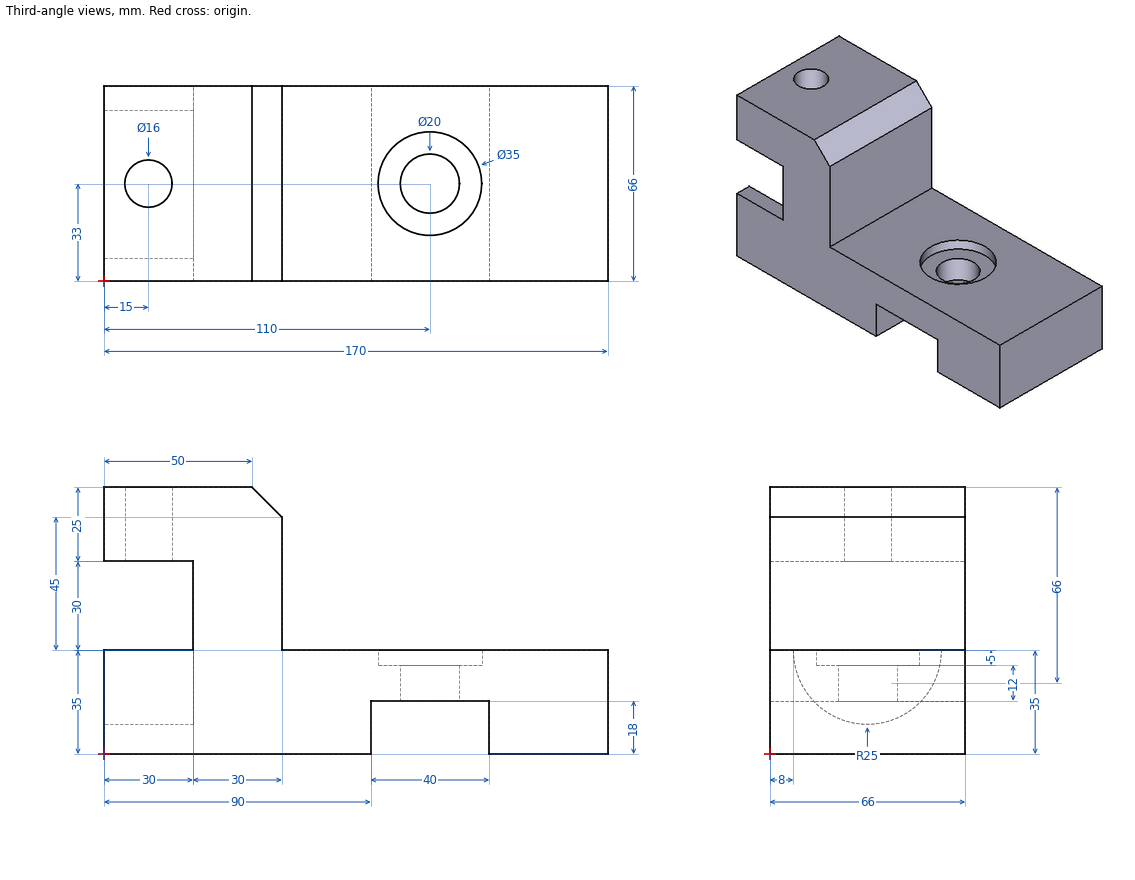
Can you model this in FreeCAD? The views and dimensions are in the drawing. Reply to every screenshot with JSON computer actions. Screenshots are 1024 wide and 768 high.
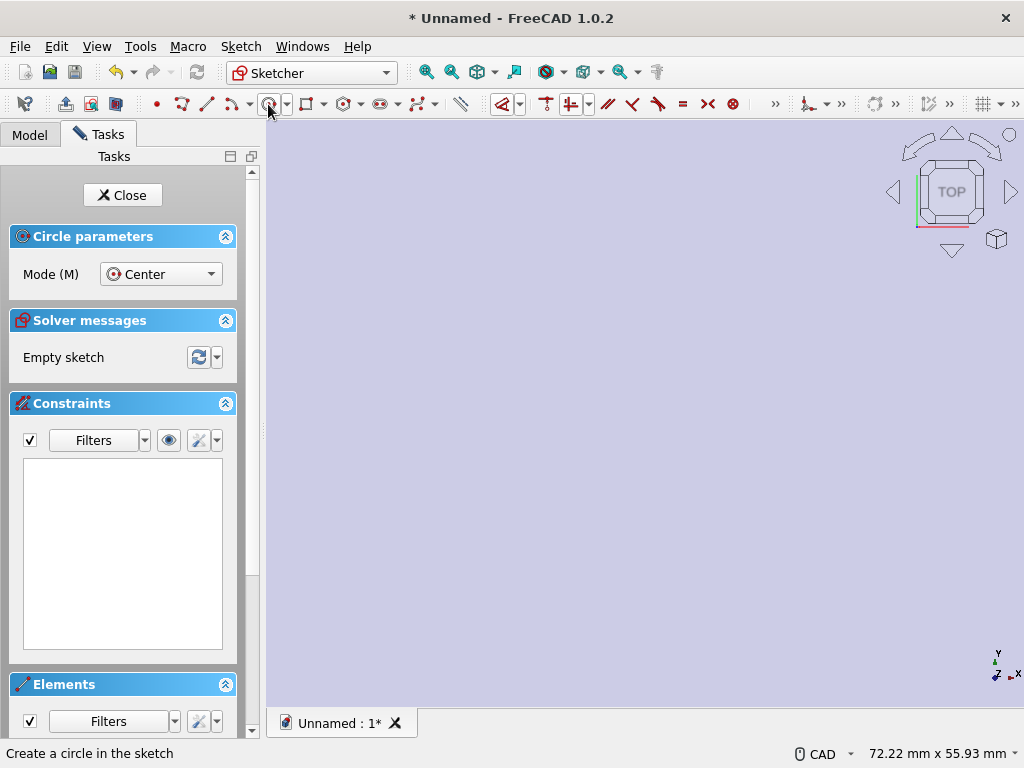
{"action": "left_click", "coordinate": [574, 411]}
{"action": "mouse_move", "coordinate": [704, 281]}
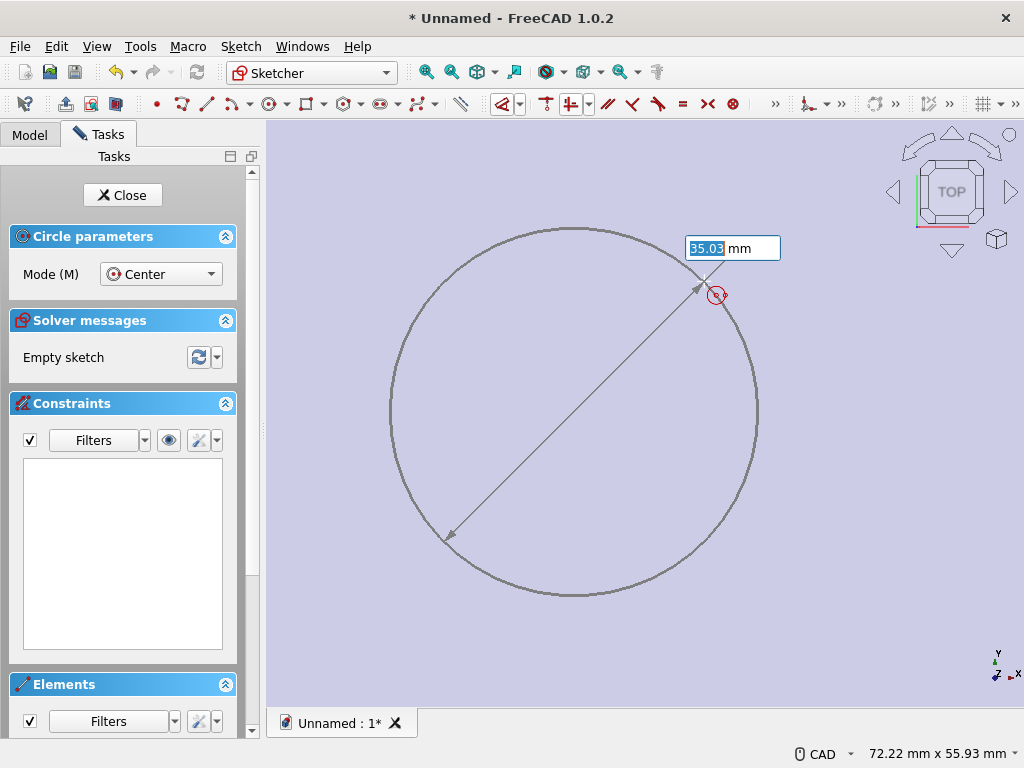
{"action": "type", "text": "35"}
{"action": "key", "text": "Return"}
{"action": "key", "text": "Escape"}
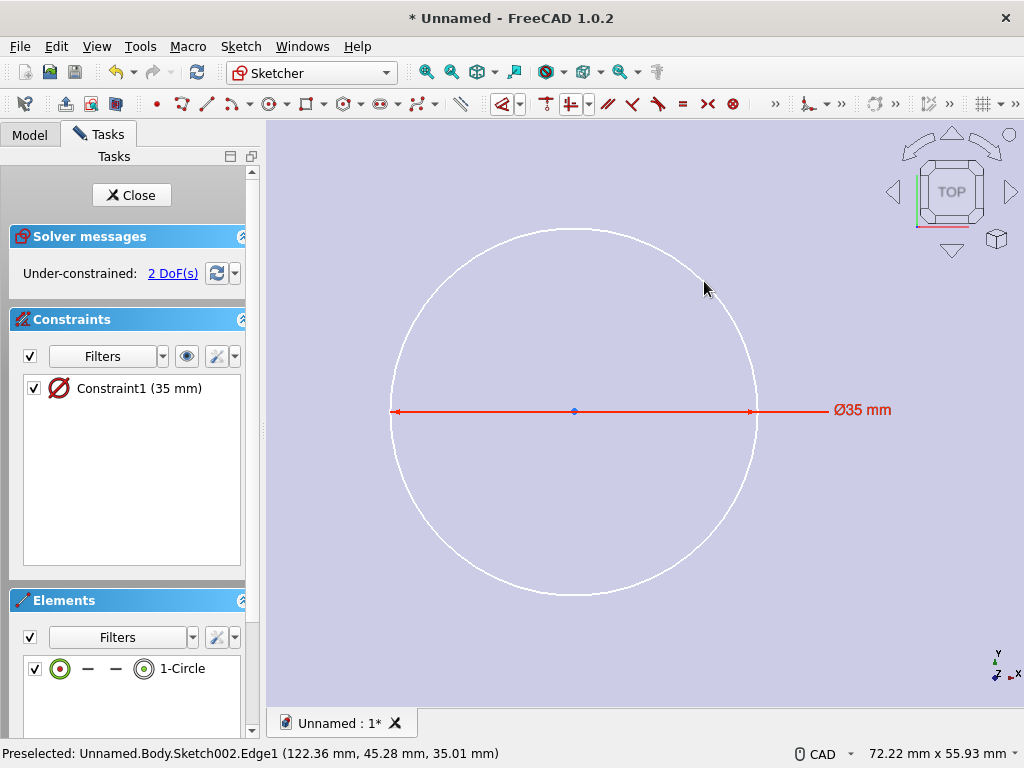
{"action": "left_click", "coordinate": [574, 412]}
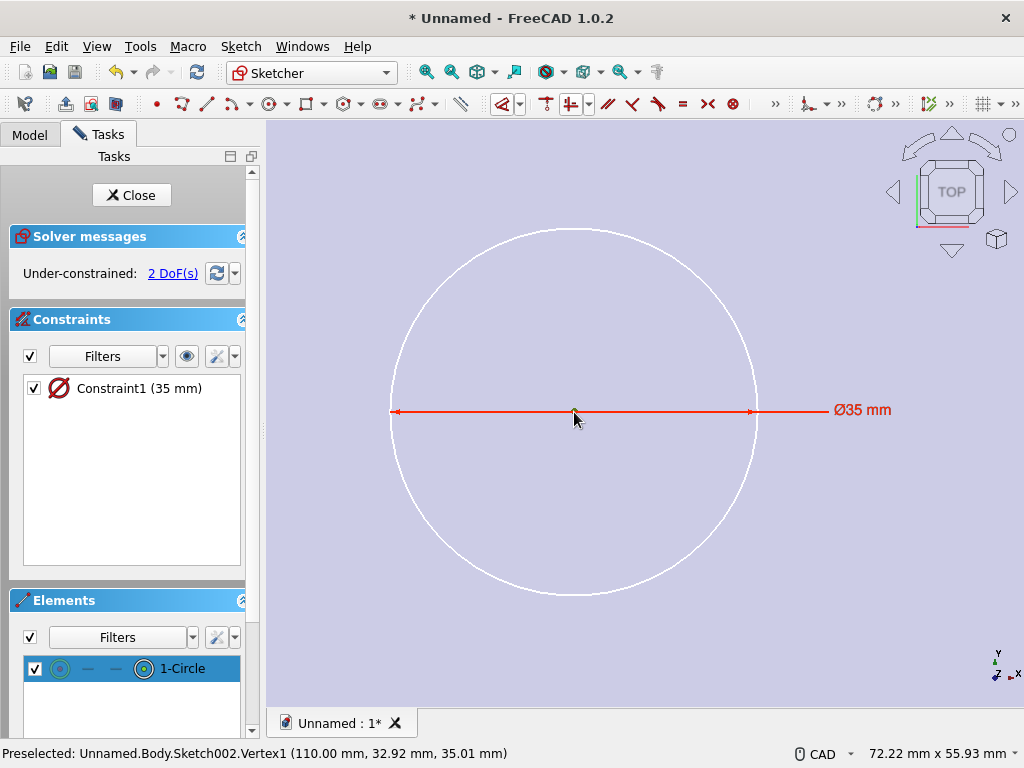
{"action": "key", "text": "i"}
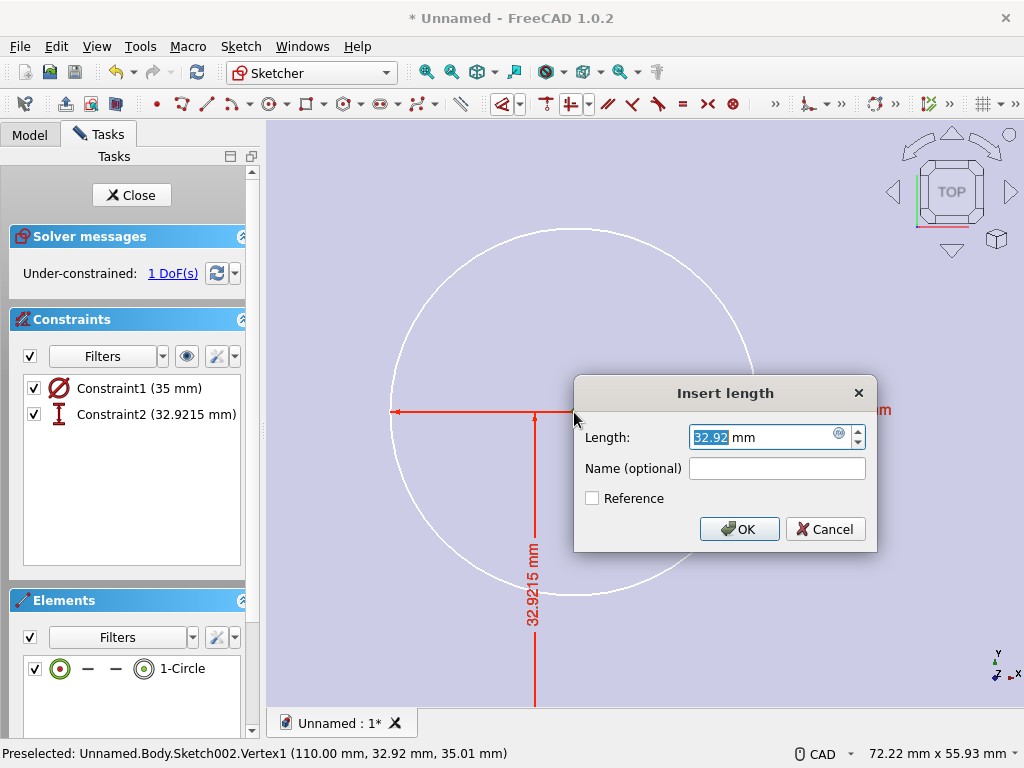
{"action": "type", "text": "33"}
{"action": "key", "text": "Return"}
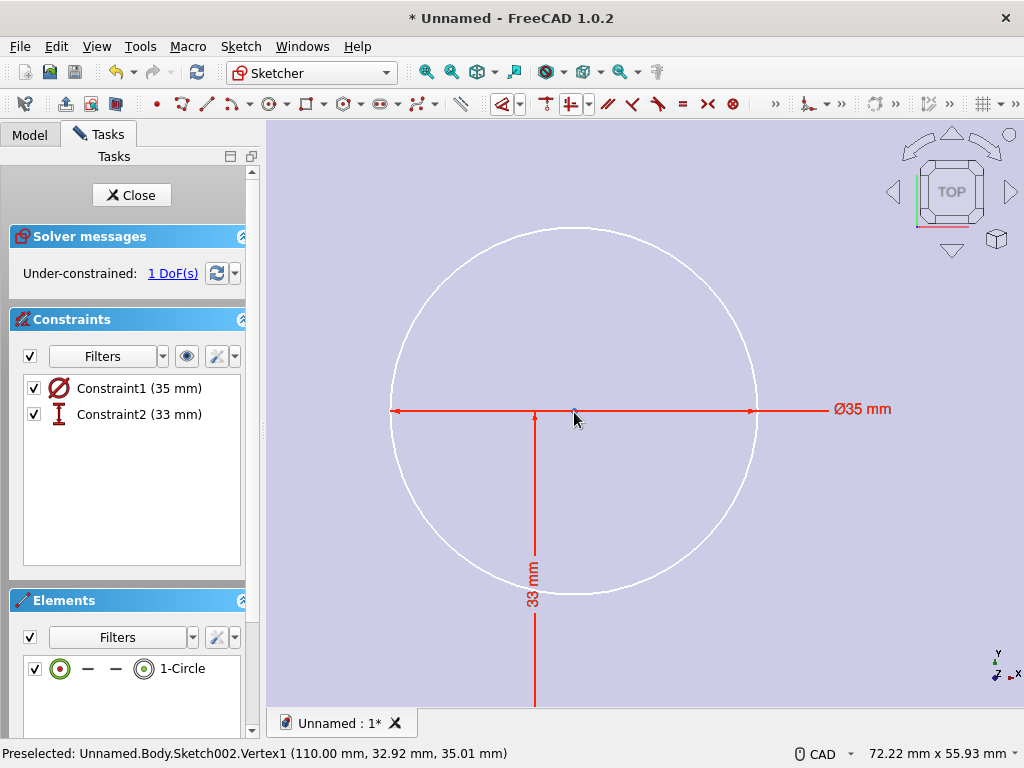
{"action": "left_click", "coordinate": [574, 411]}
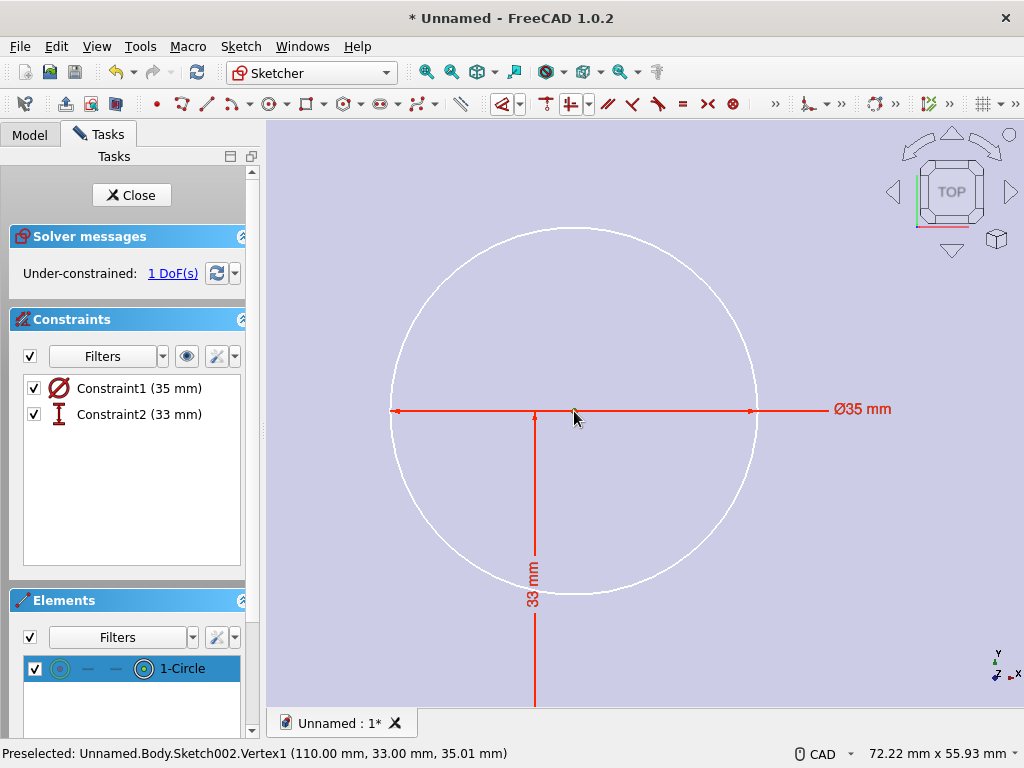
{"action": "left_click", "coordinate": [520, 104]}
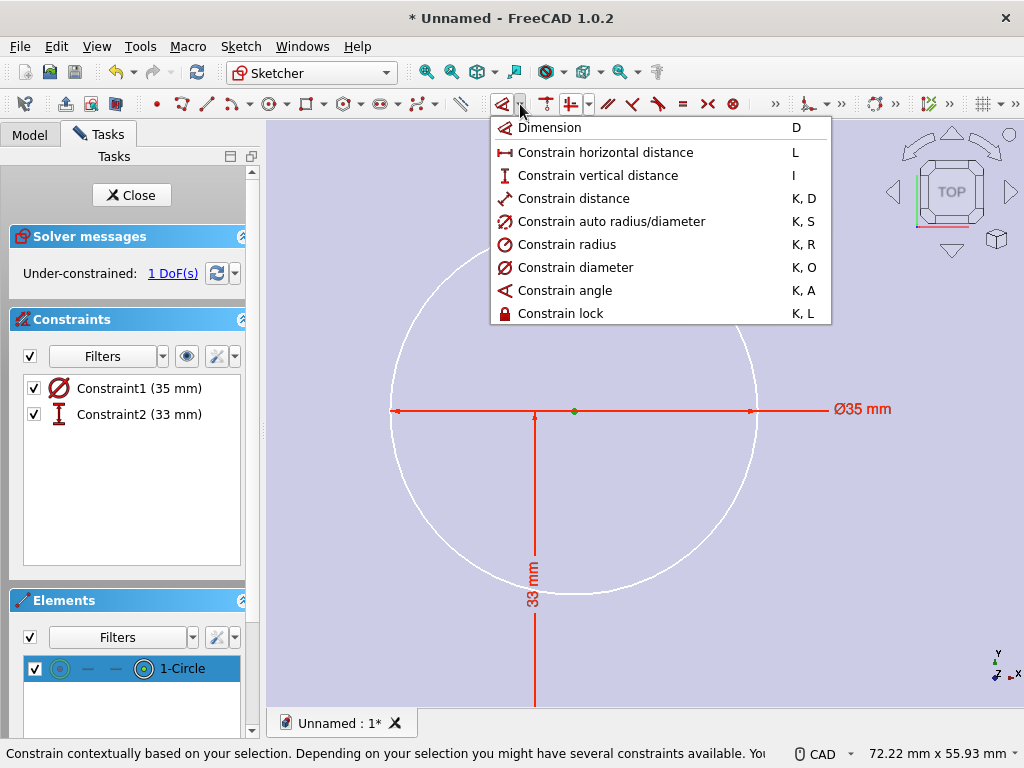
{"action": "left_click", "coordinate": [661, 152]}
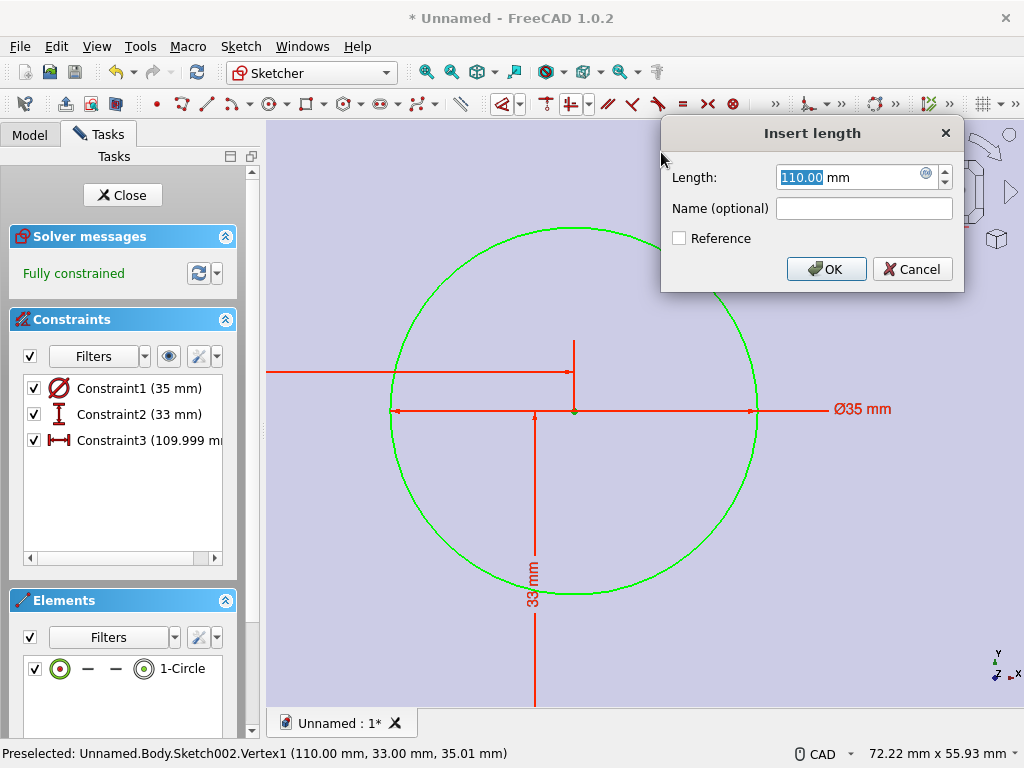
{"action": "type", "text": "110"}
{"action": "key", "text": "Return"}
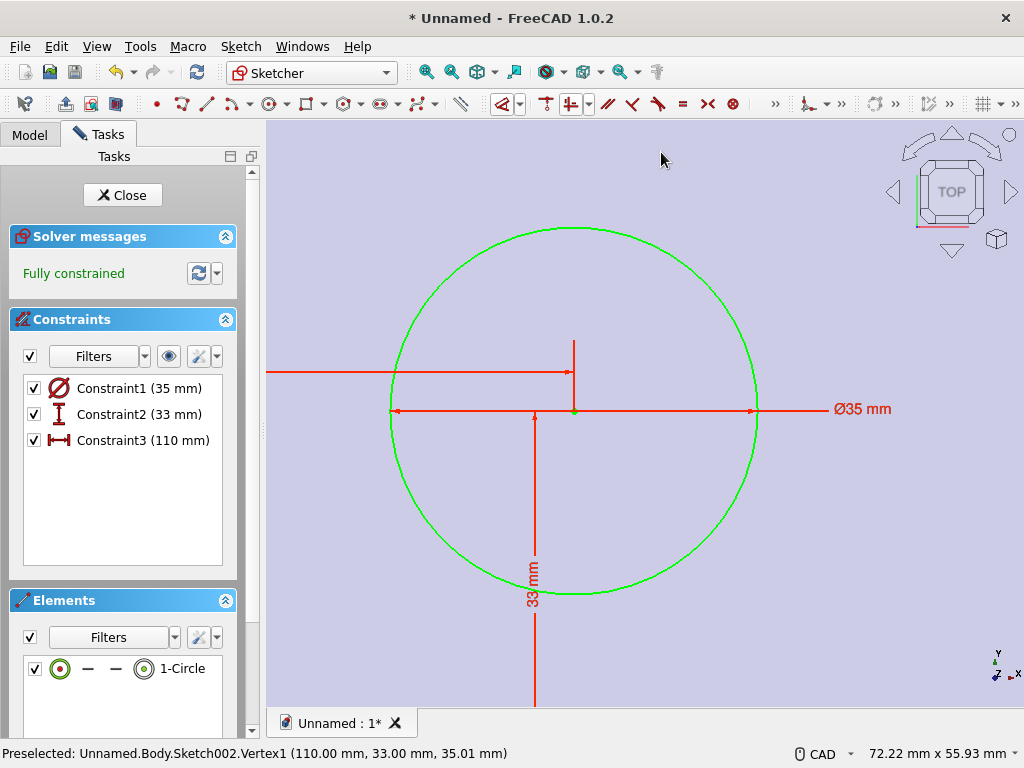
{"action": "left_click", "coordinate": [123, 195]}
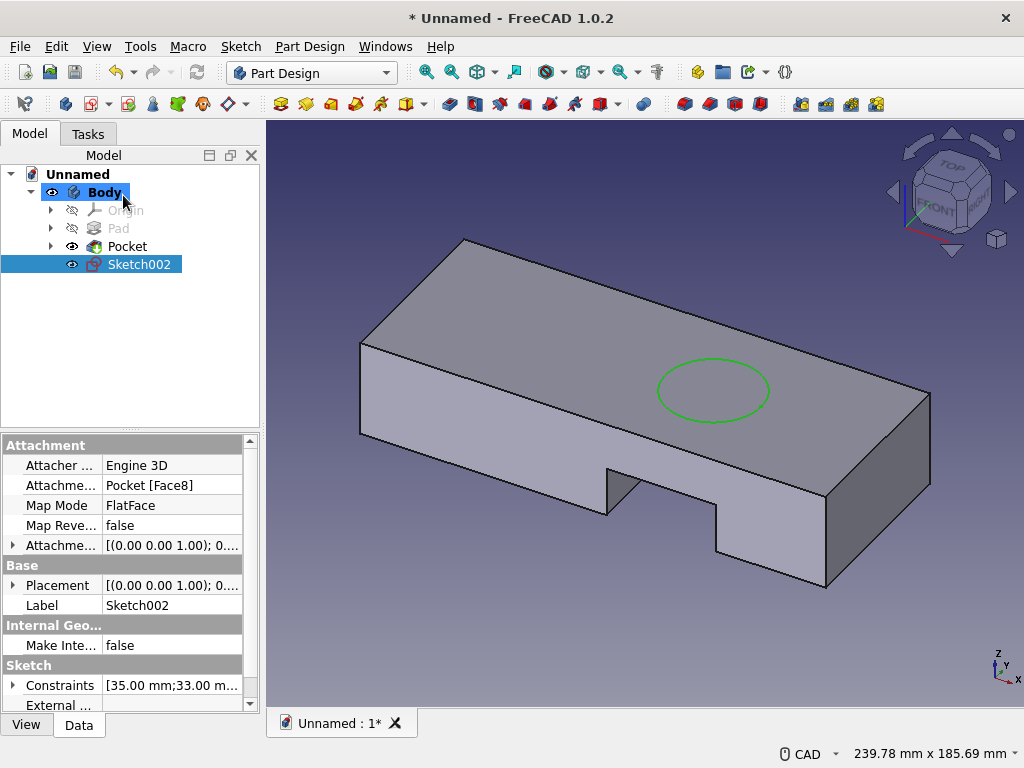
{"action": "left_click", "coordinate": [450, 104]}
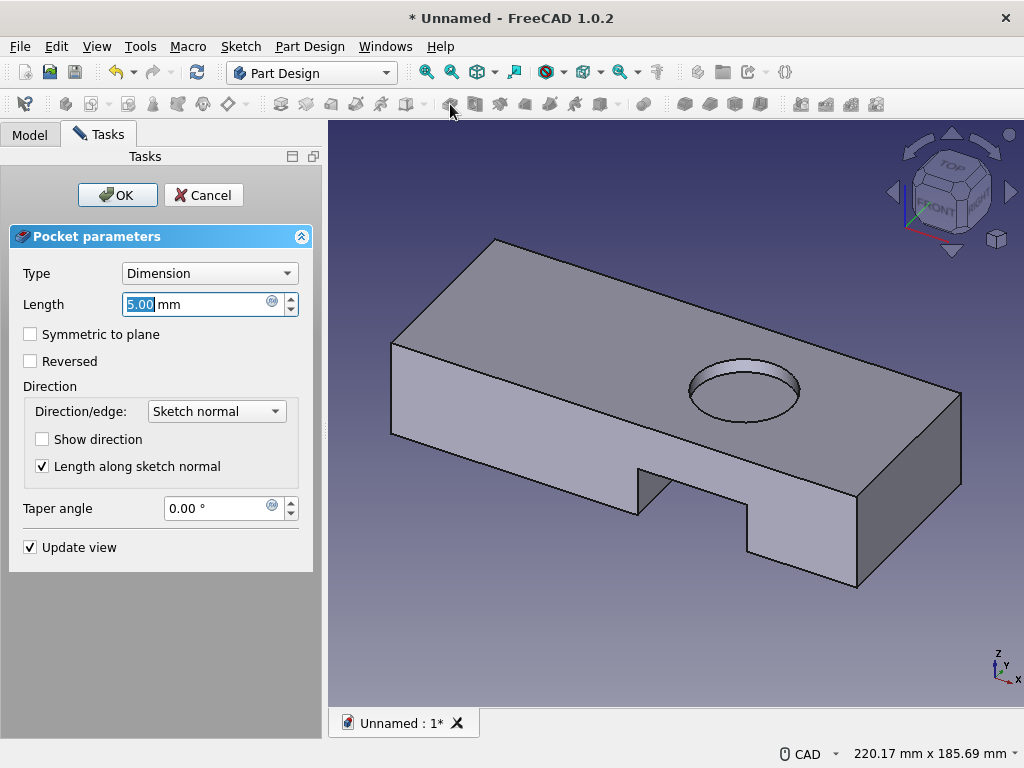
{"action": "type", "text": "5"}
{"action": "key", "text": "Tab"}